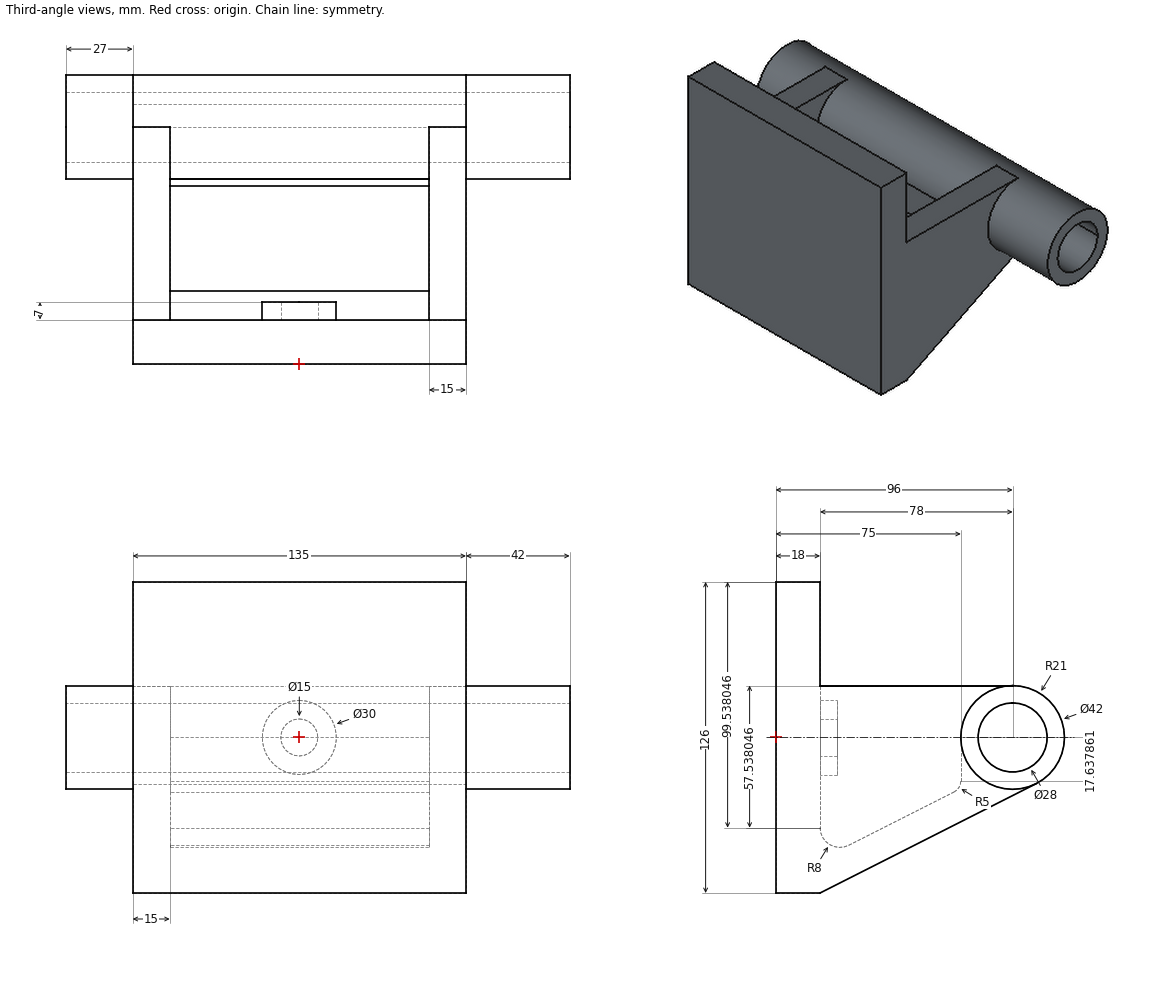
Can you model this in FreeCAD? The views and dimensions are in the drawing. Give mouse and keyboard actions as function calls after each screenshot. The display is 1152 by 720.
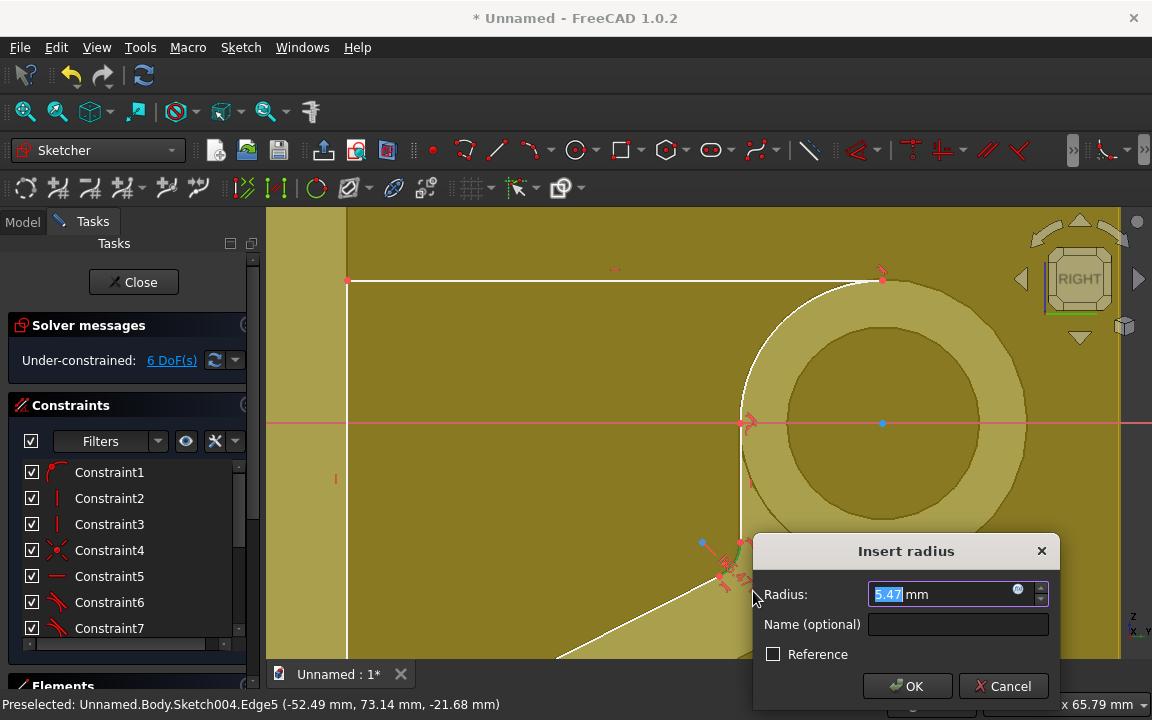
text(5)
key(Return)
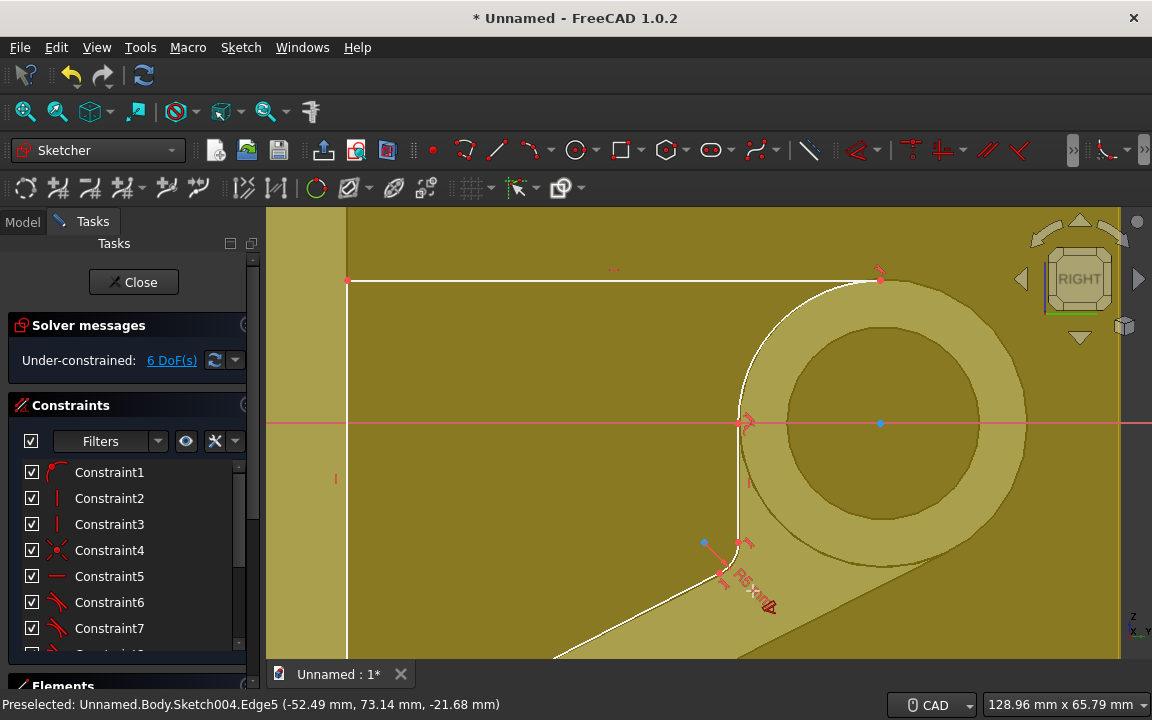
scroll(817, 295, down, 2)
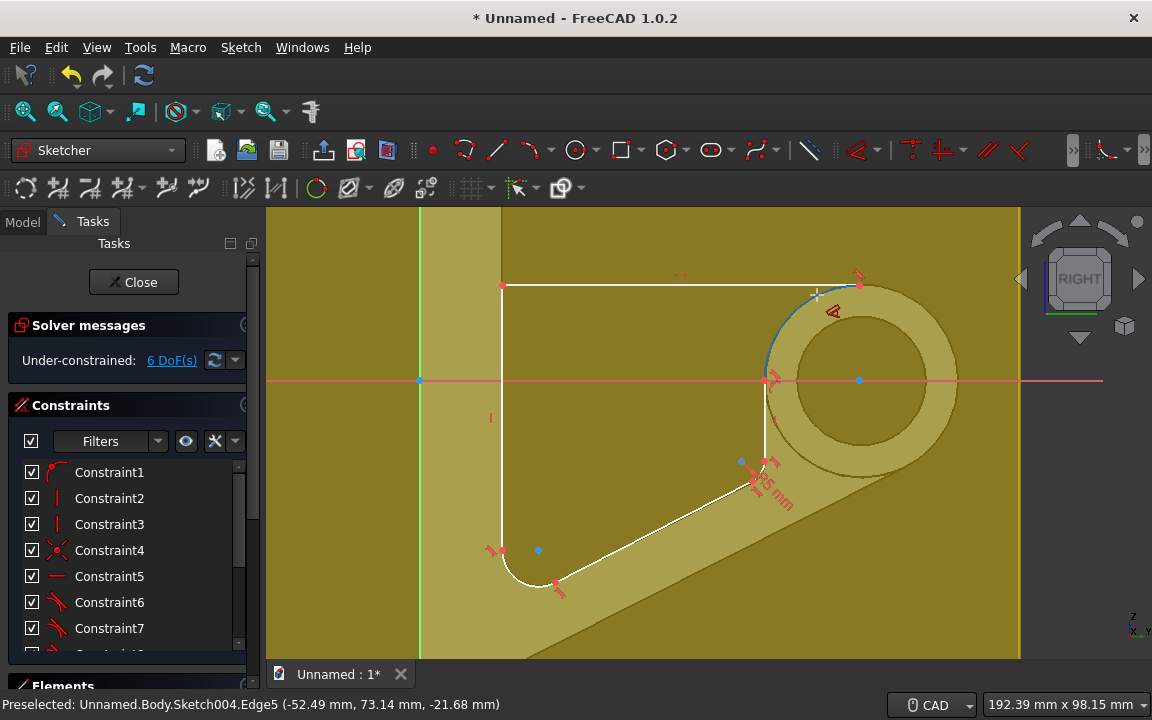
click(509, 571)
click(483, 589)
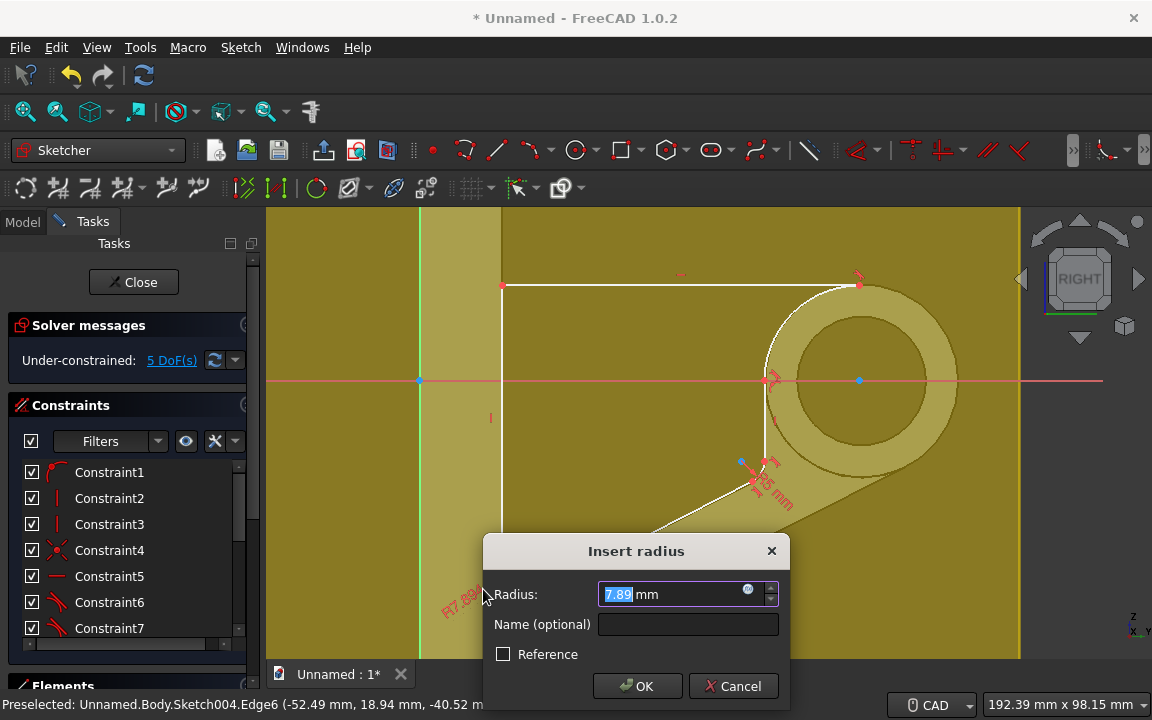
text(8)
key(Return)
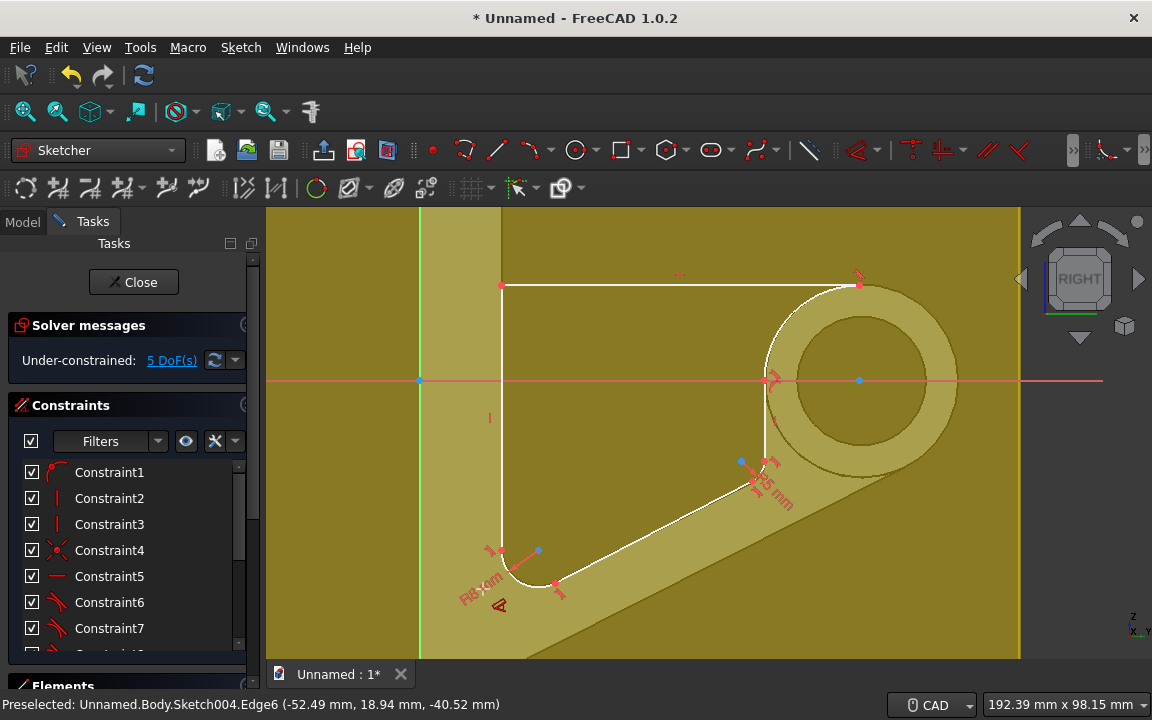
scroll(817, 296, up, 2)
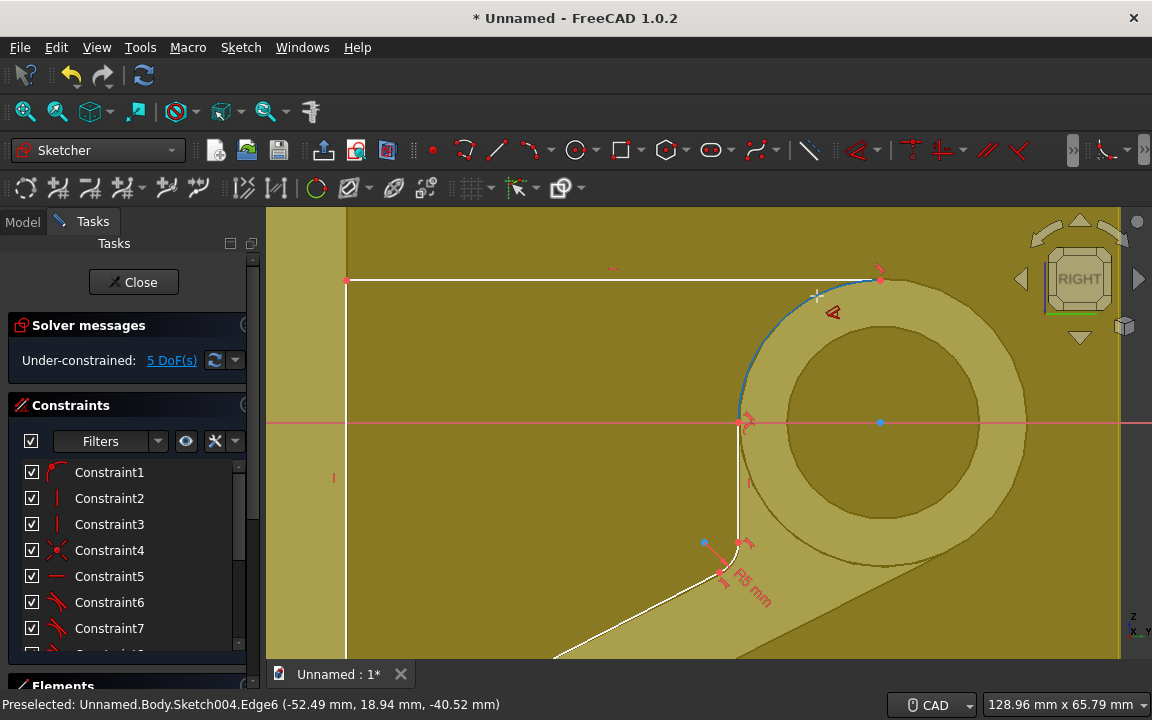
click(816, 296)
click(886, 248)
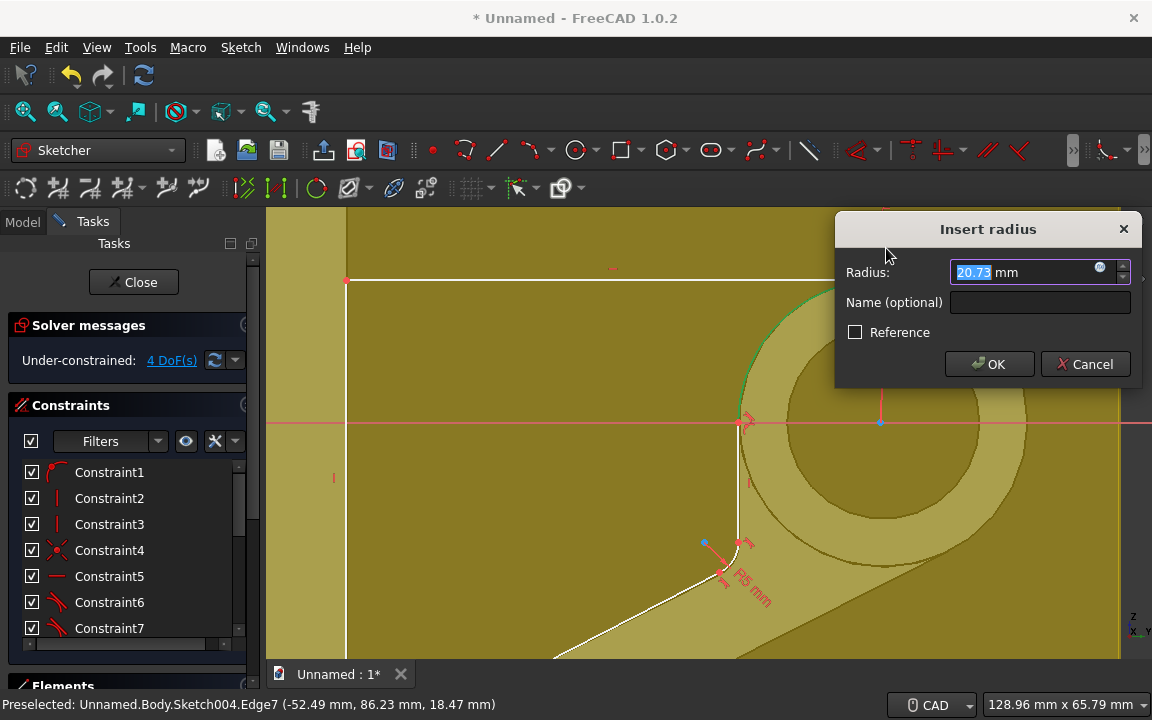
text(21)
key(Return)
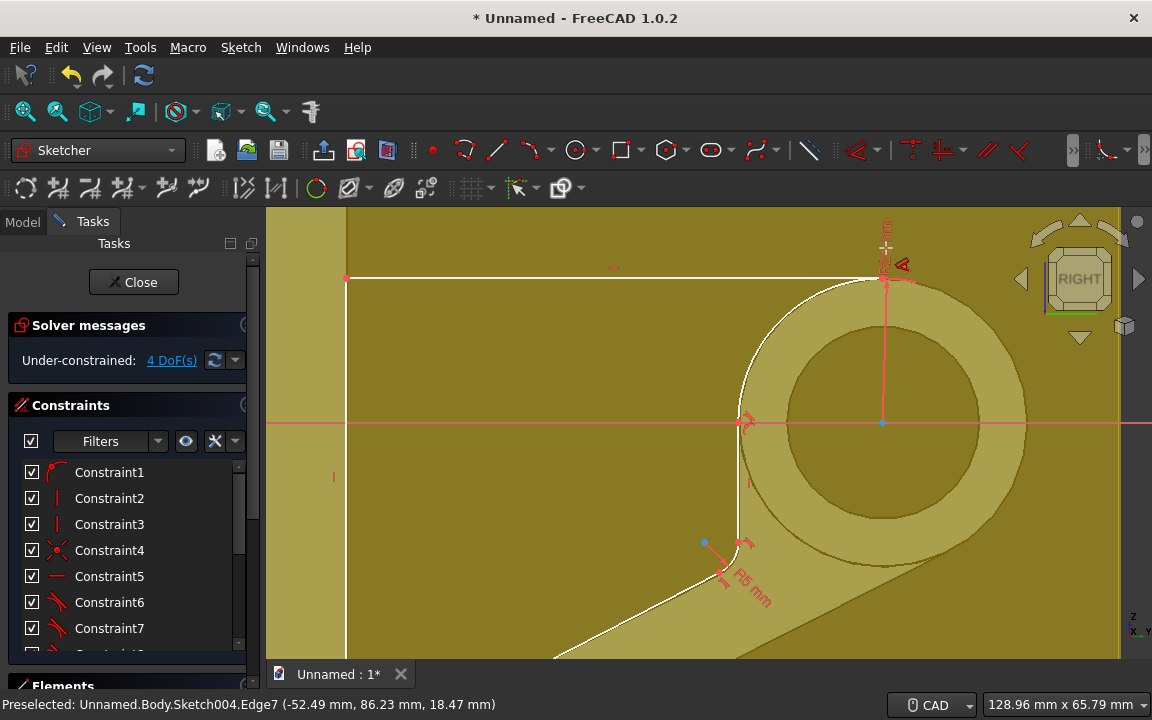
click(507, 278)
click(614, 244)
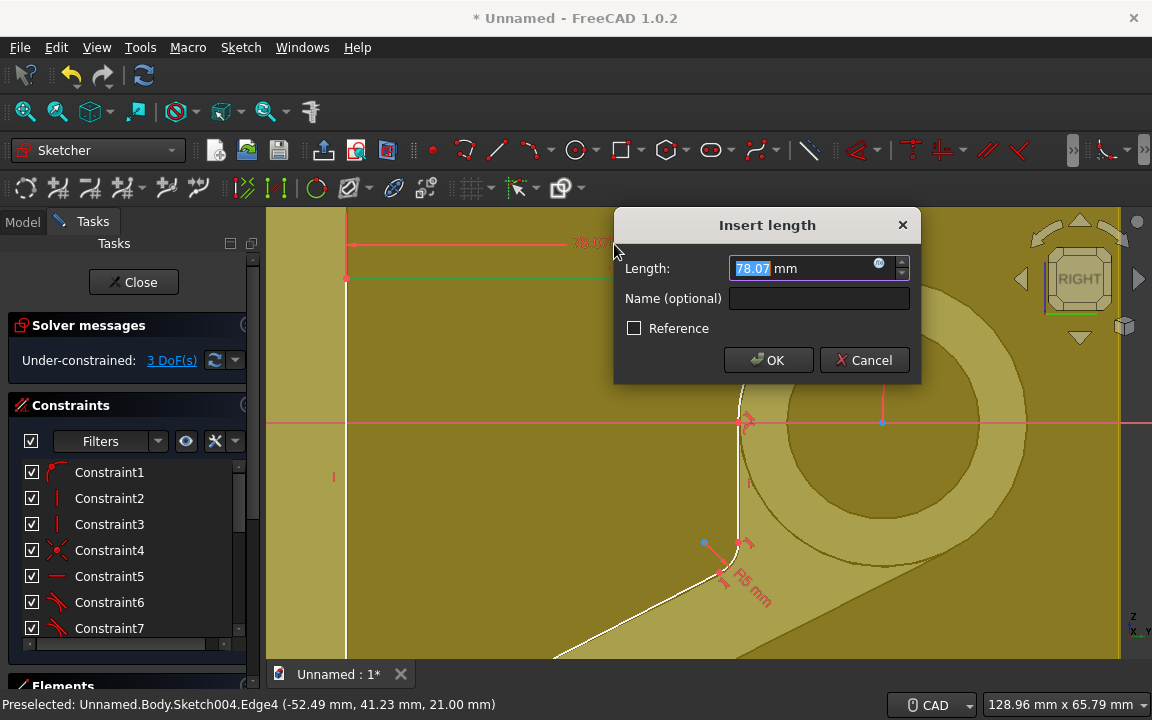
text(78)
key(Return)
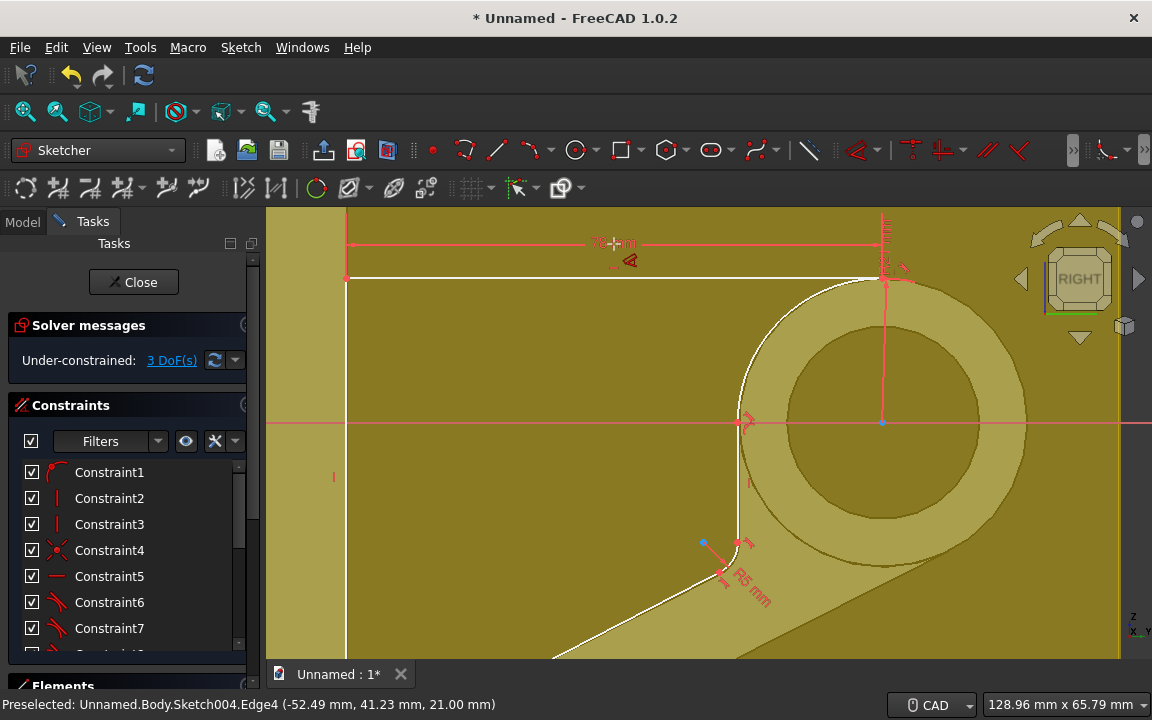
click(738, 423)
click(516, 389)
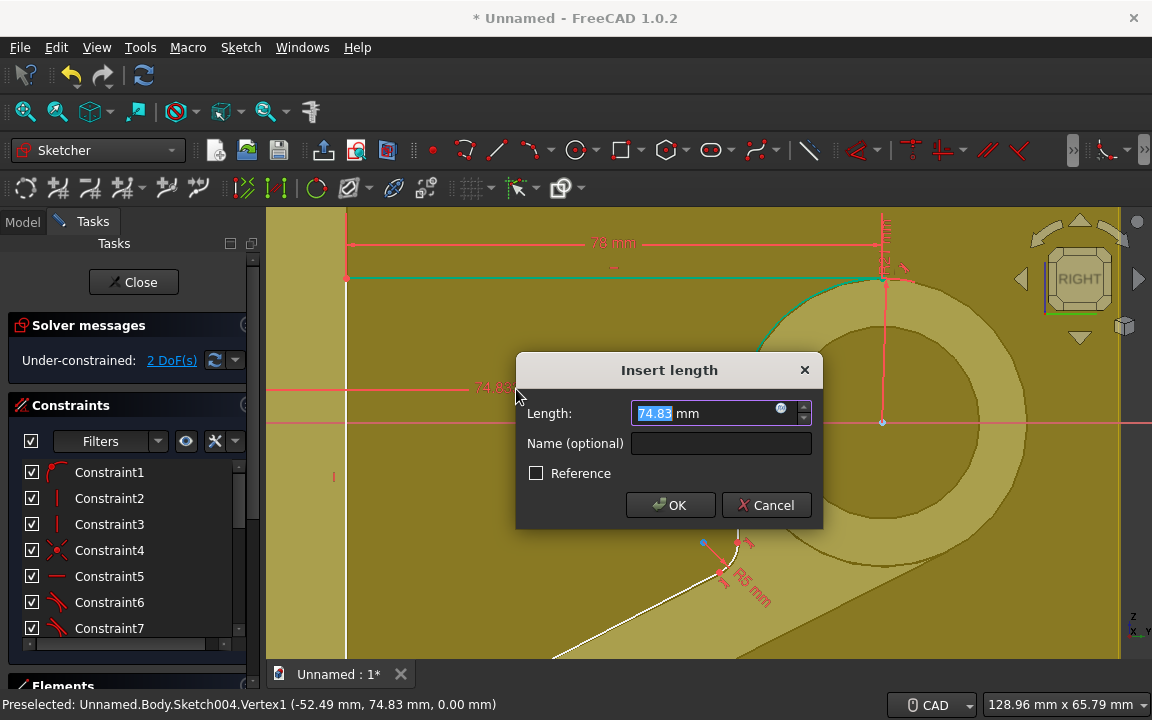
text(75)
key(Return)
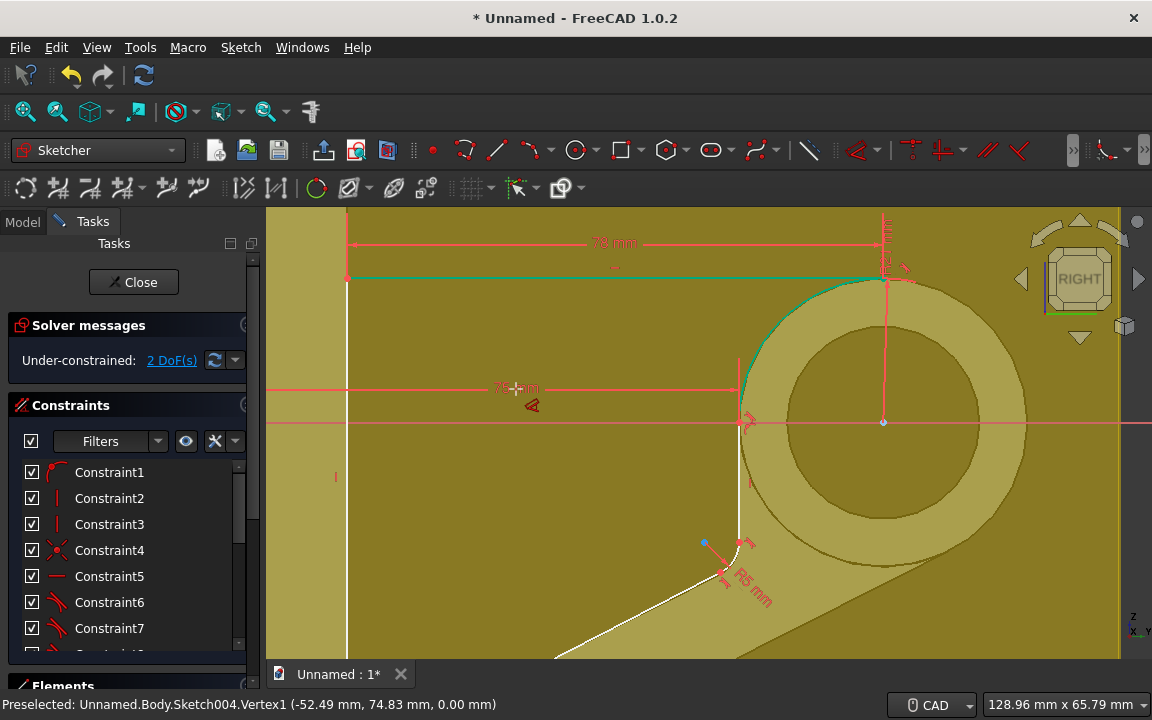
click(739, 458)
click(773, 482)